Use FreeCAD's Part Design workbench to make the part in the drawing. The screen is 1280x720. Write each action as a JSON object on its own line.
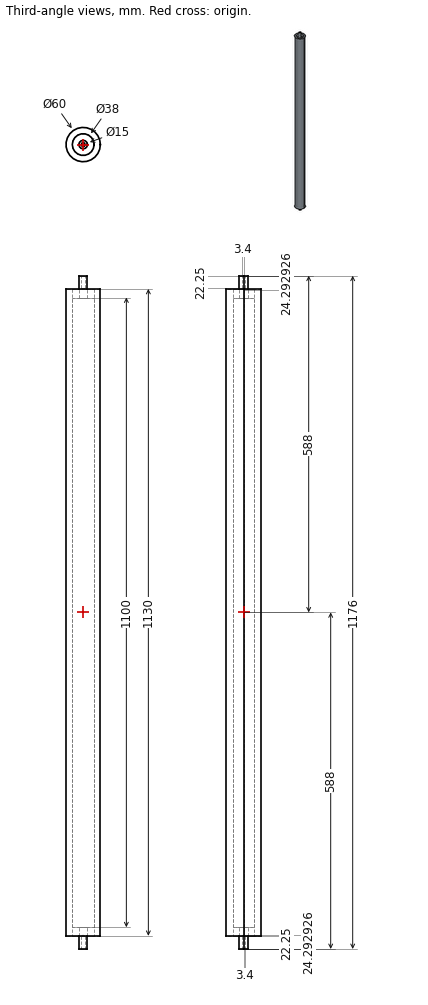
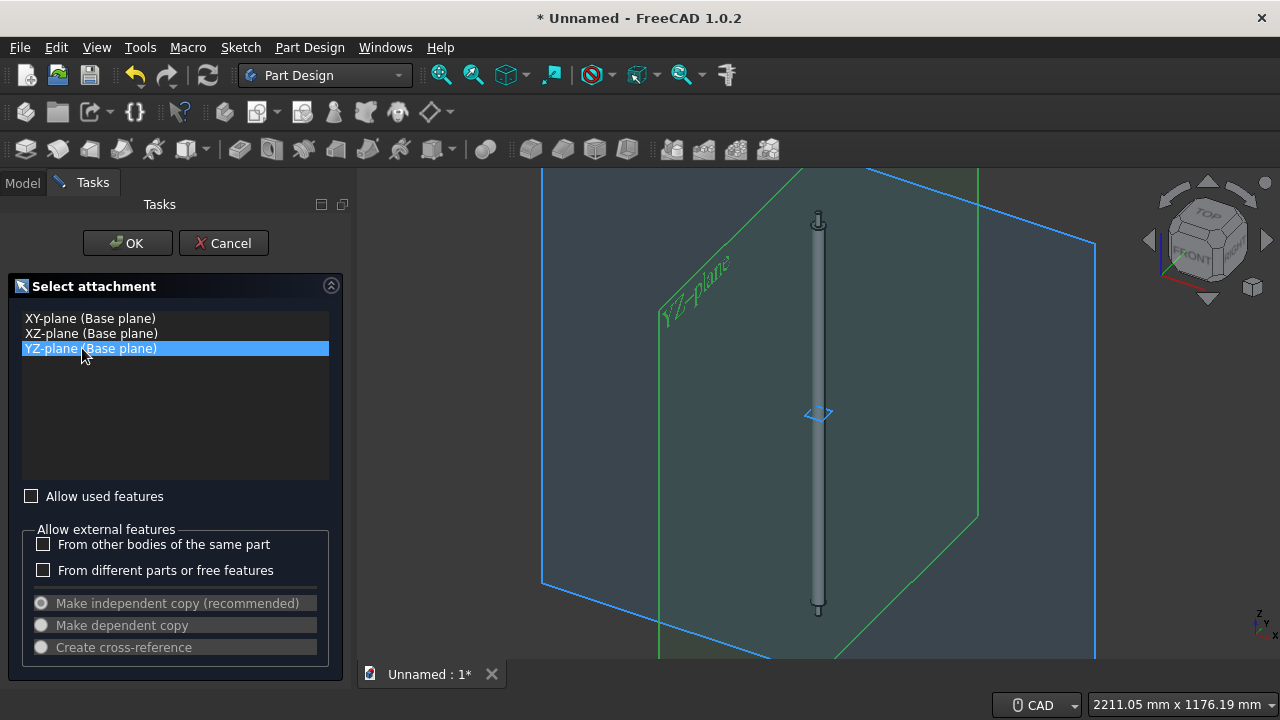
{"action": "left_click", "coordinate": [128, 243]}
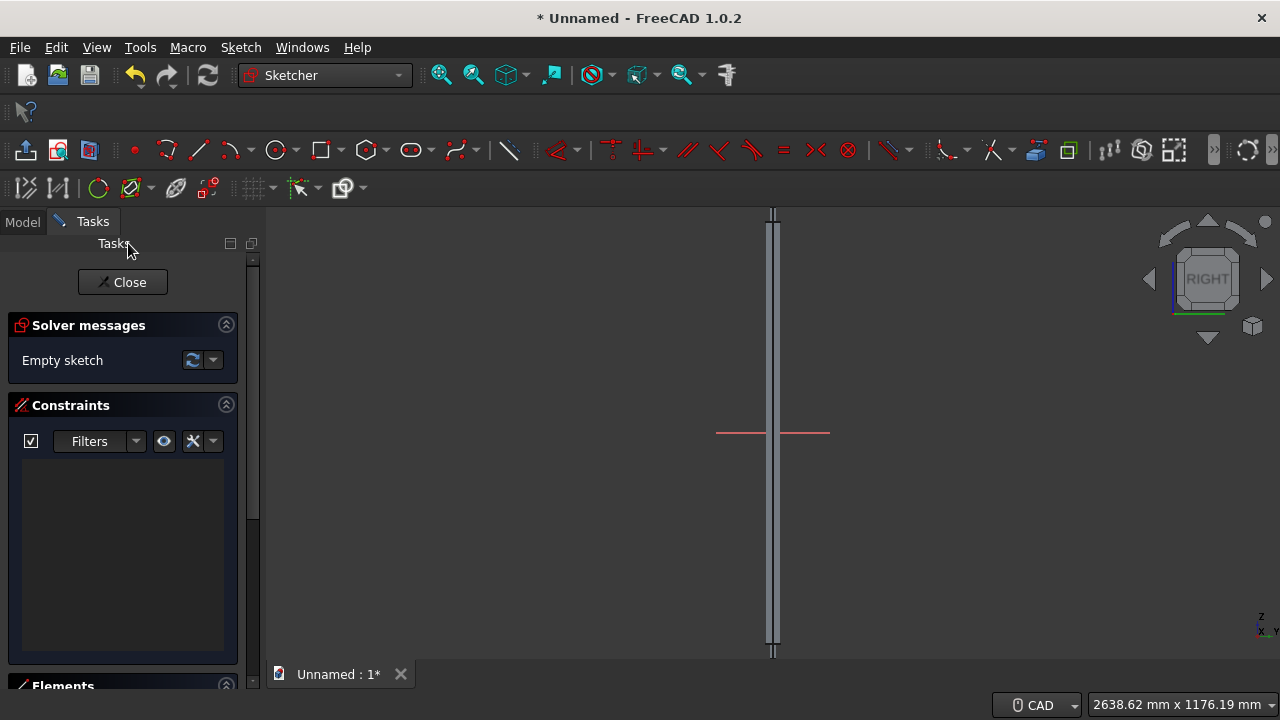
{"action": "left_click", "coordinate": [90, 150]}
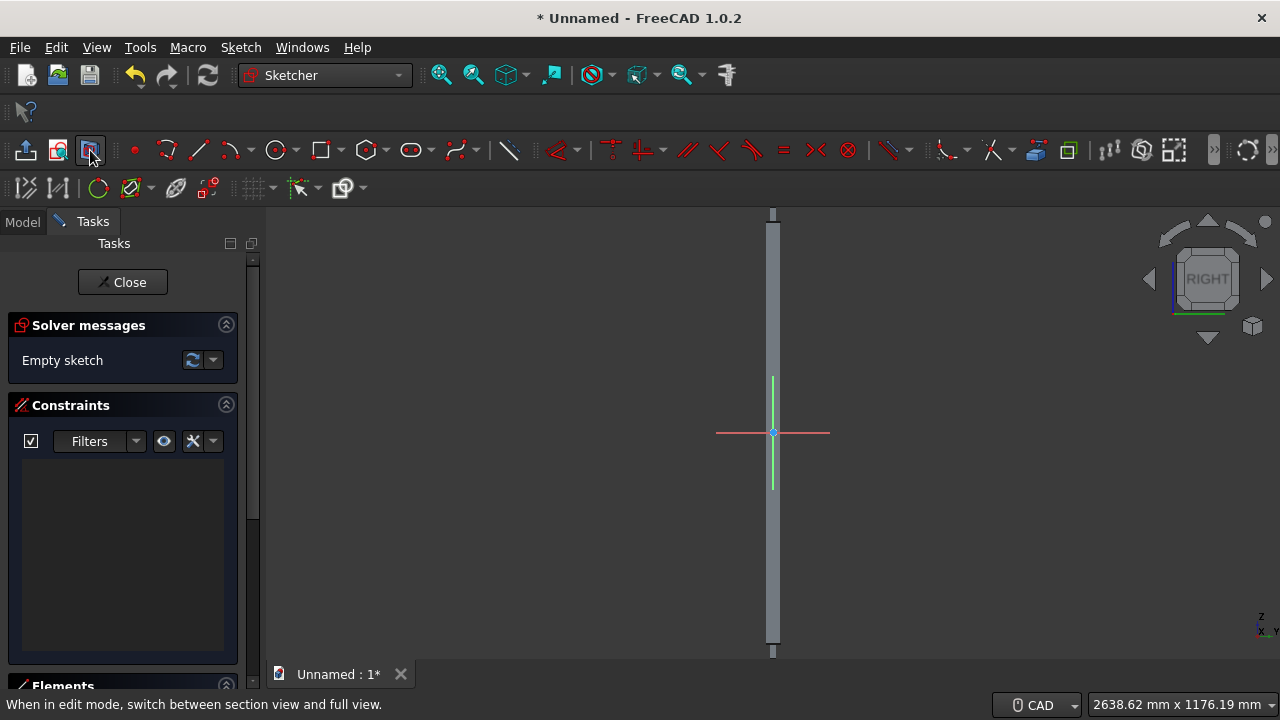
{"action": "scroll", "coordinate": [704, 433], "scroll_direction": "down", "scroll_amount": 5}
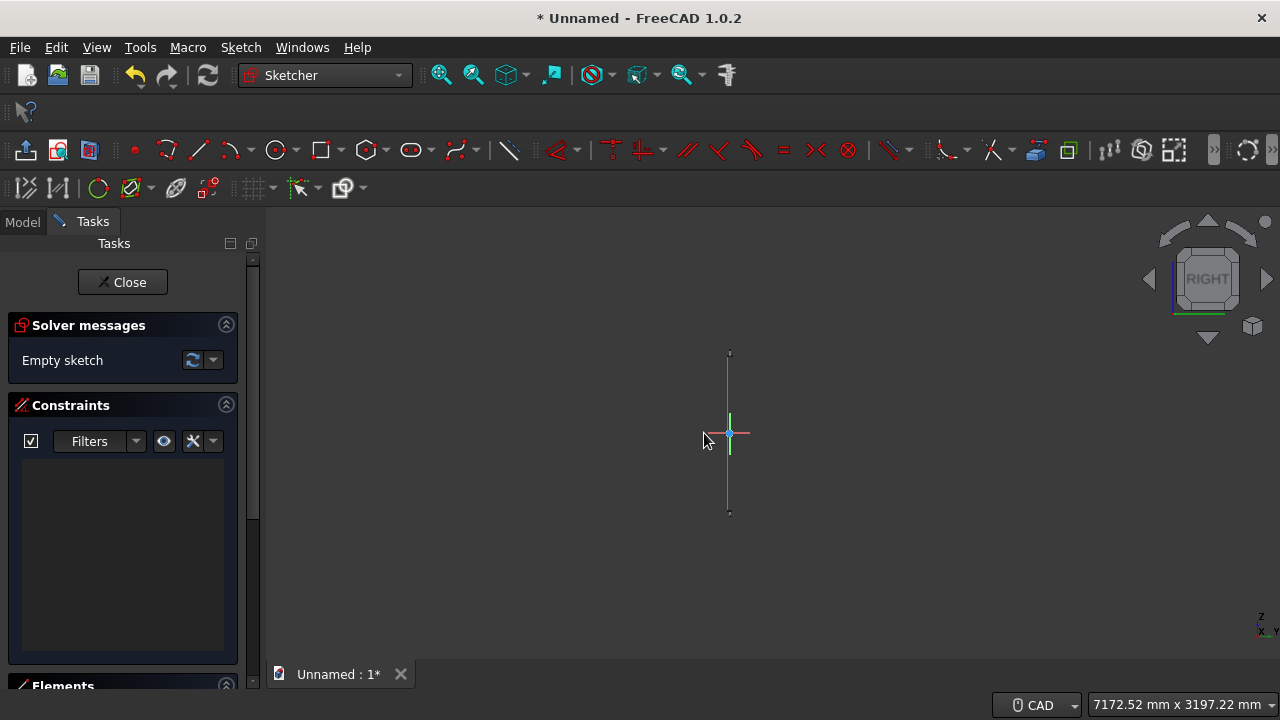
{"action": "scroll", "coordinate": [731, 519], "scroll_direction": "up", "scroll_amount": 15}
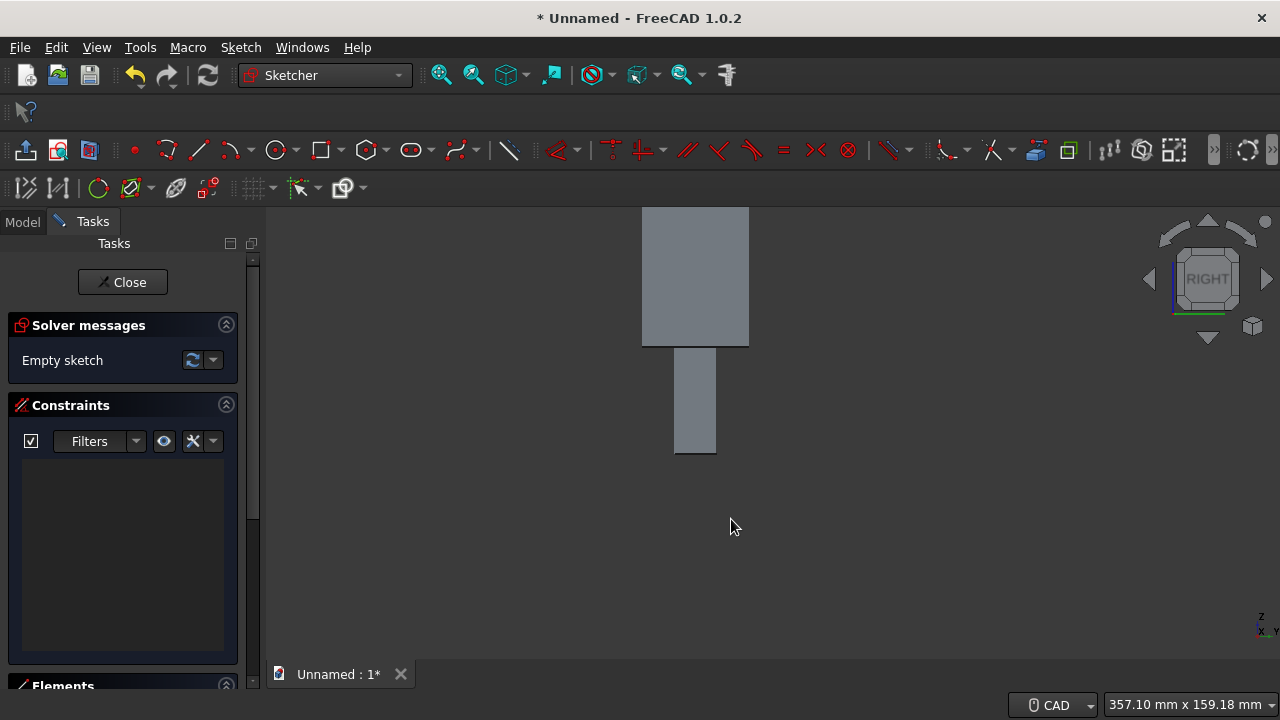
{"action": "scroll", "coordinate": [699, 416], "scroll_direction": "up", "scroll_amount": 7}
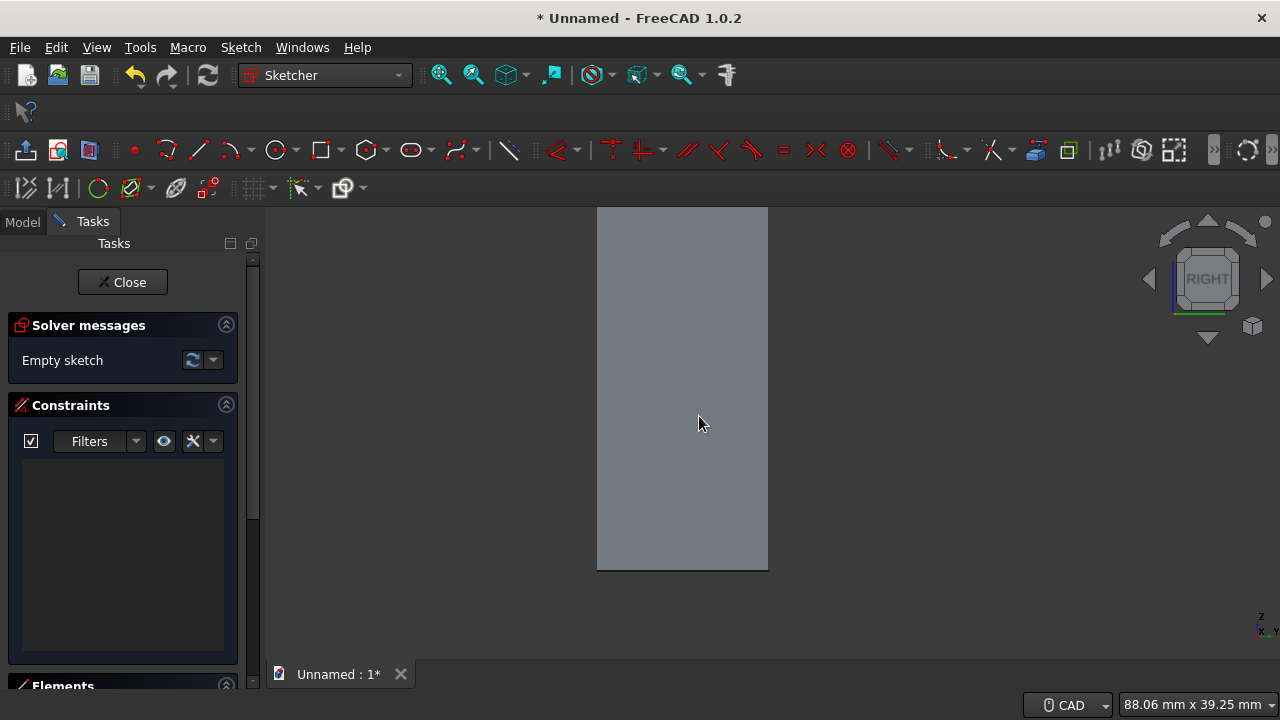
{"action": "key", "text": "g m"}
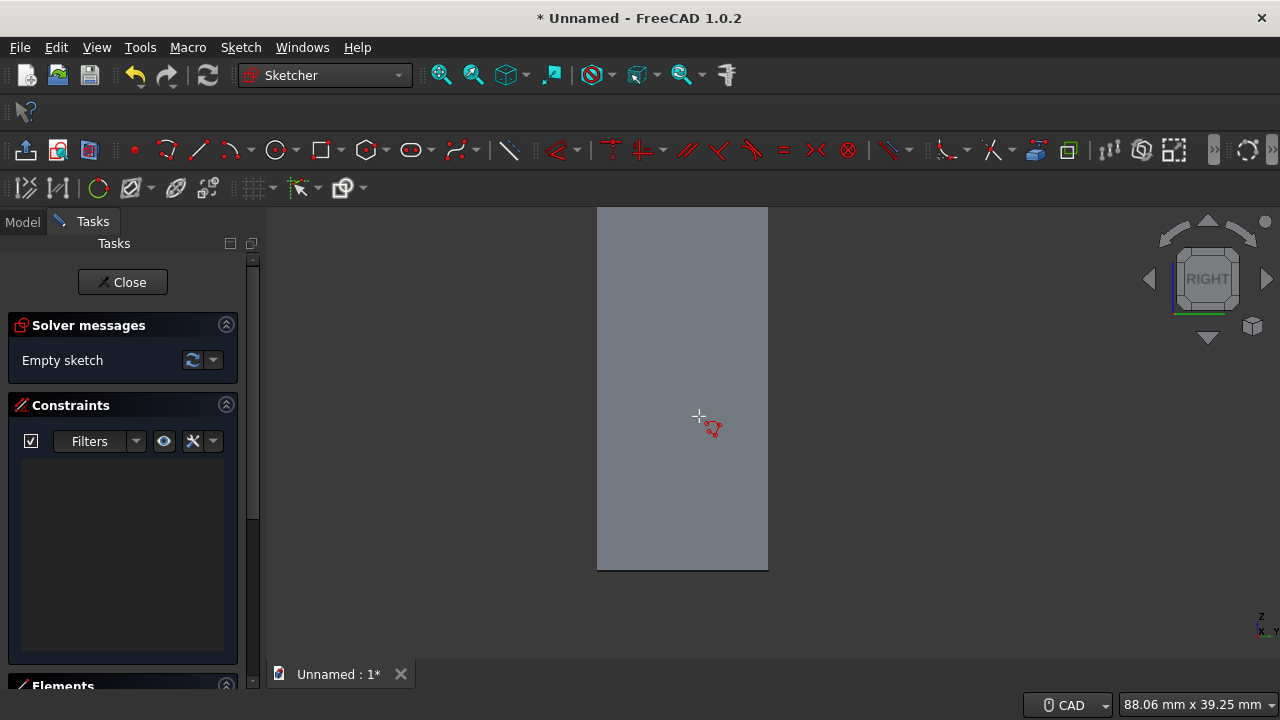
{"action": "left_click", "coordinate": [683, 291]}
{"action": "left_click", "coordinate": [692, 571]}
{"action": "left_click", "coordinate": [722, 571]}
{"action": "left_click", "coordinate": [722, 314]}
{"action": "left_click", "coordinate": [683, 292]}
{"action": "key", "text": "Escape"}
{"action": "key", "text": "Escape"}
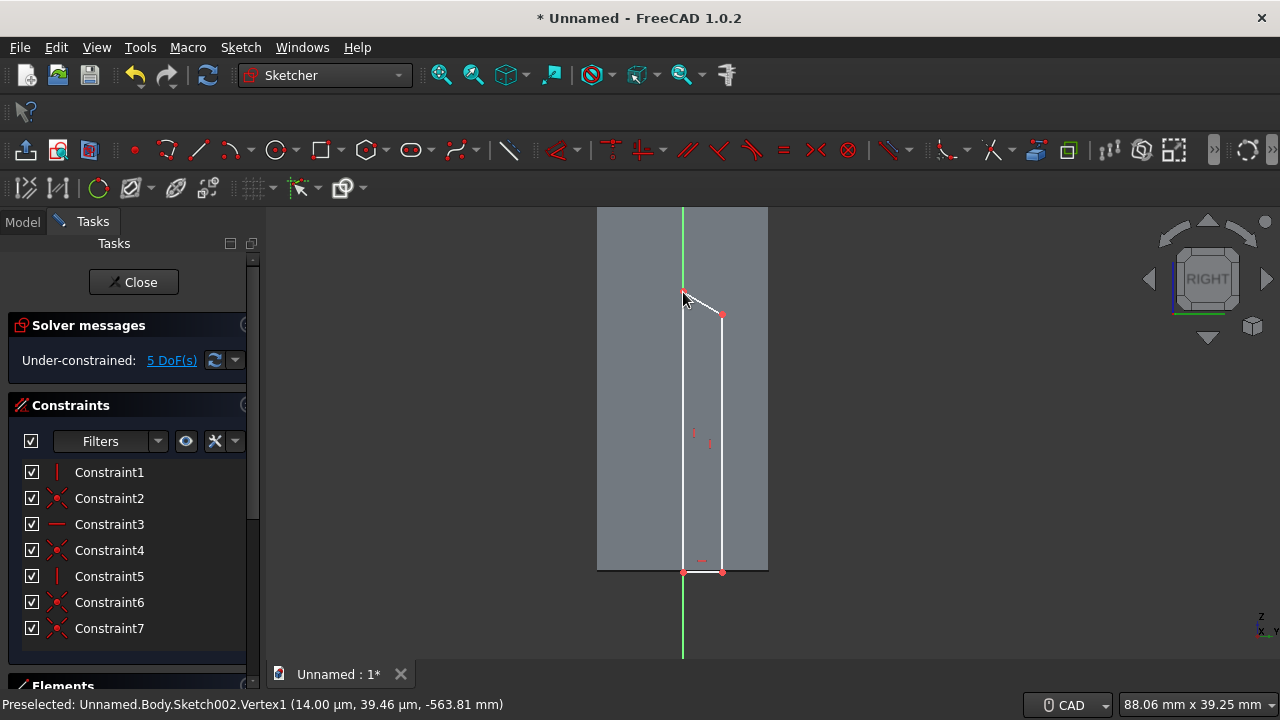
{"action": "left_click", "coordinate": [683, 292]}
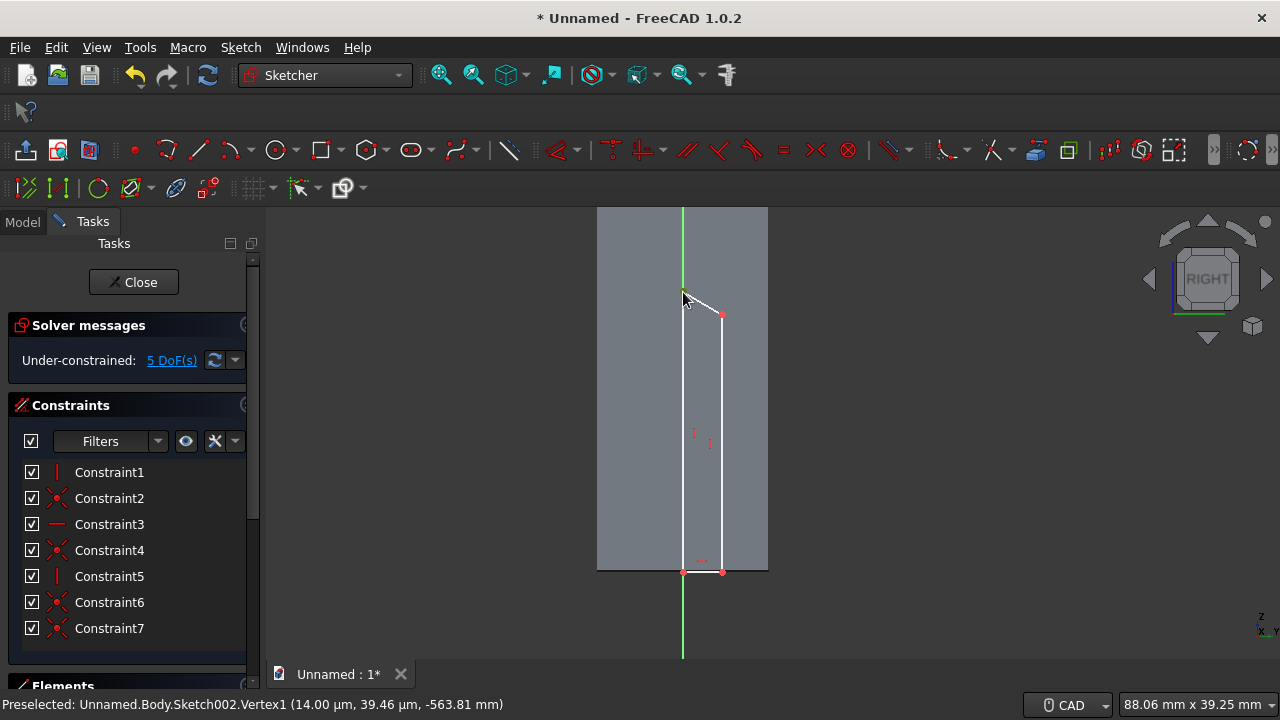
{"action": "left_click", "coordinate": [683, 603]}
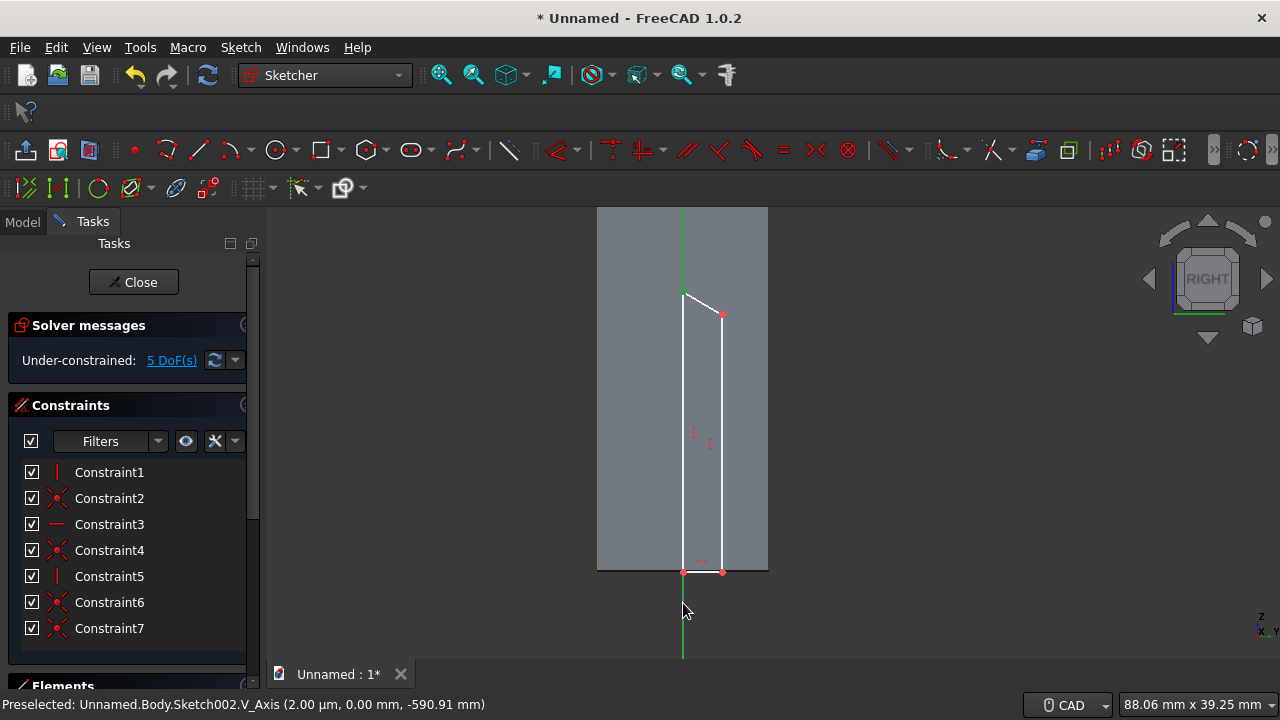
{"action": "key", "text": "c"}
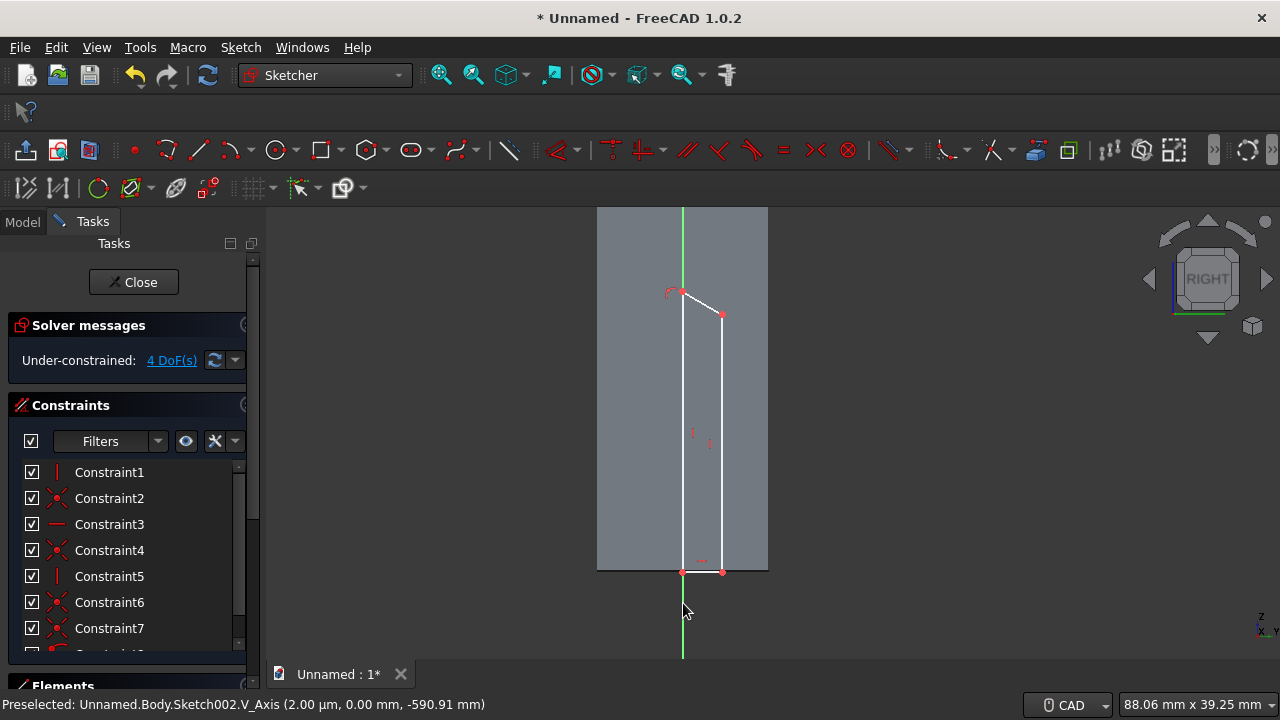
{"action": "left_click", "coordinate": [556, 150]}